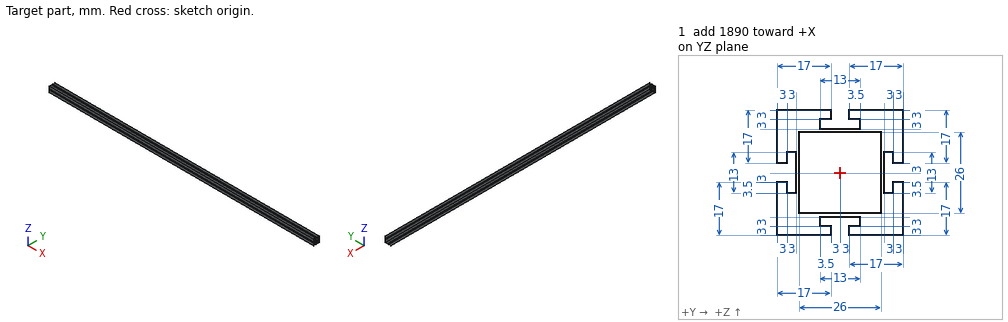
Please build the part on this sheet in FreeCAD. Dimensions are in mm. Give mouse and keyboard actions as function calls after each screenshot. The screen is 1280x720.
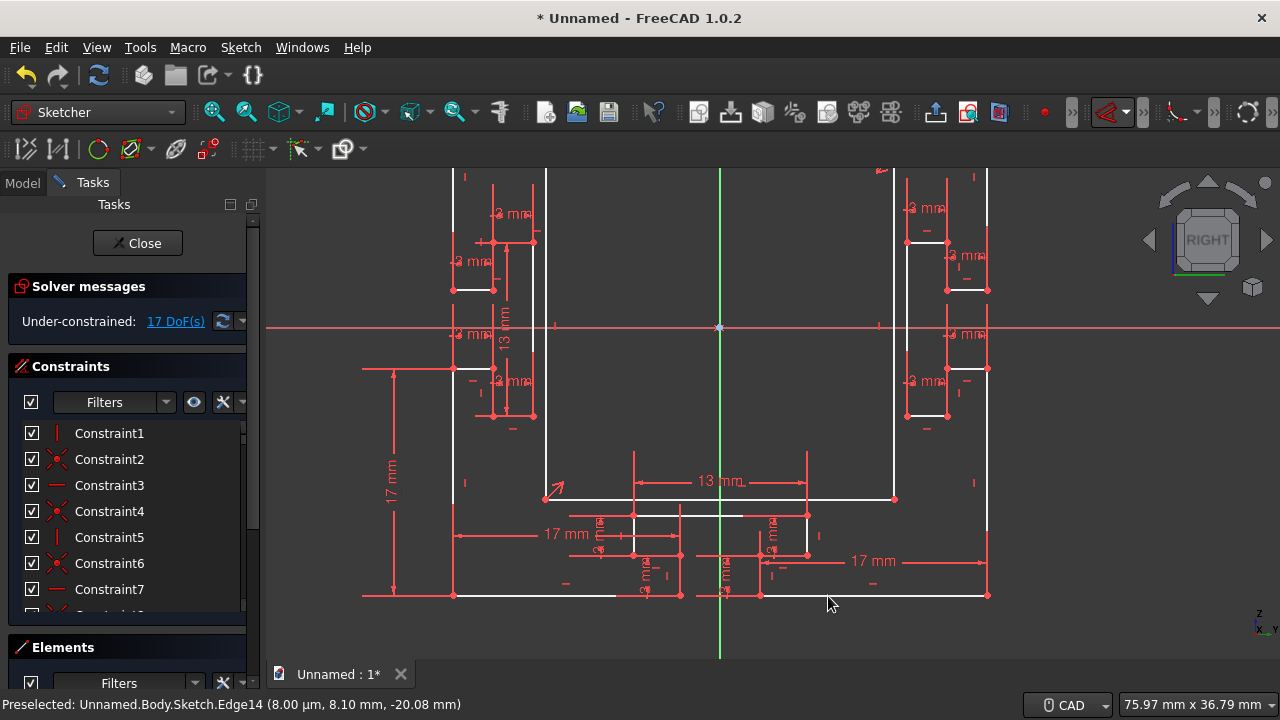
click(987, 528)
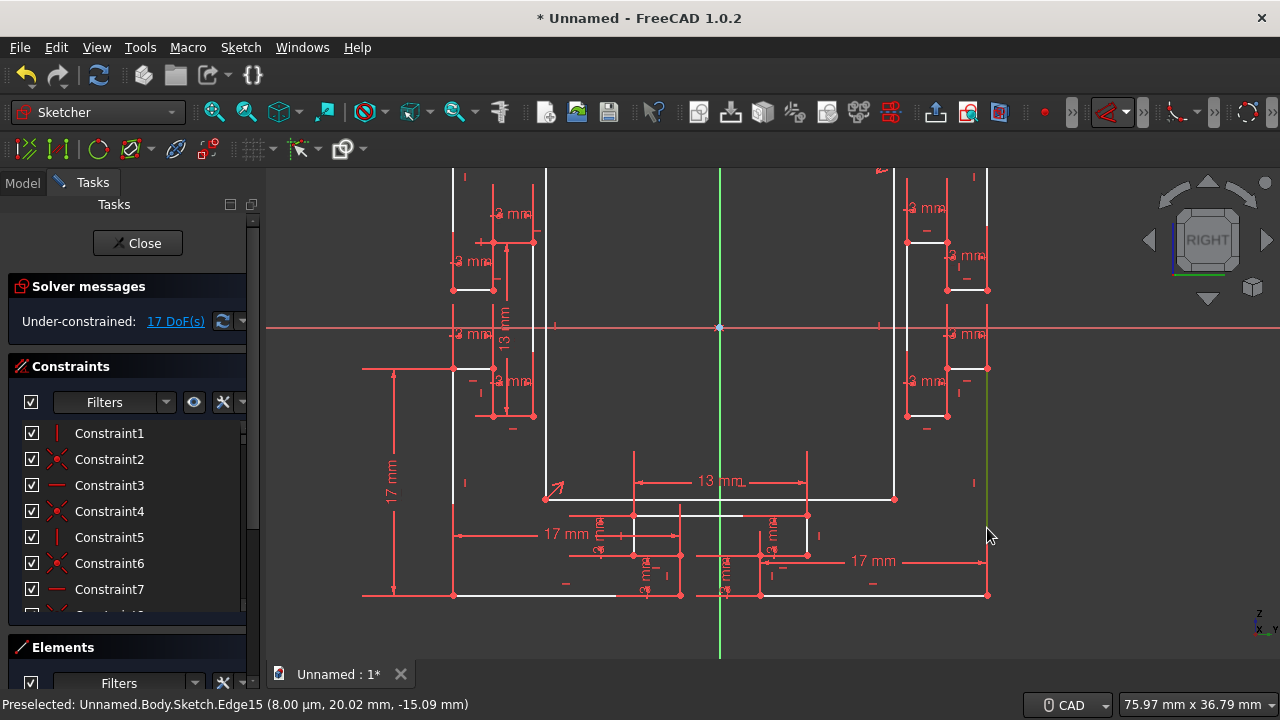
click(1128, 112)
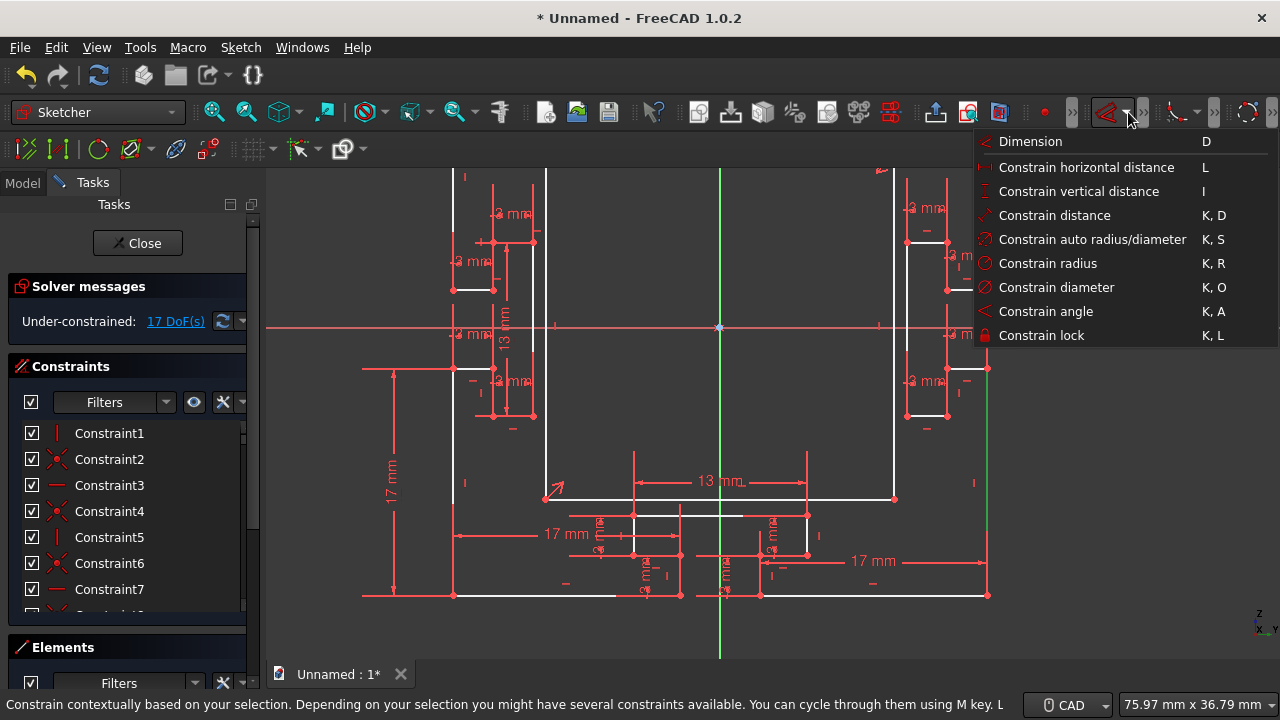
click(1126, 191)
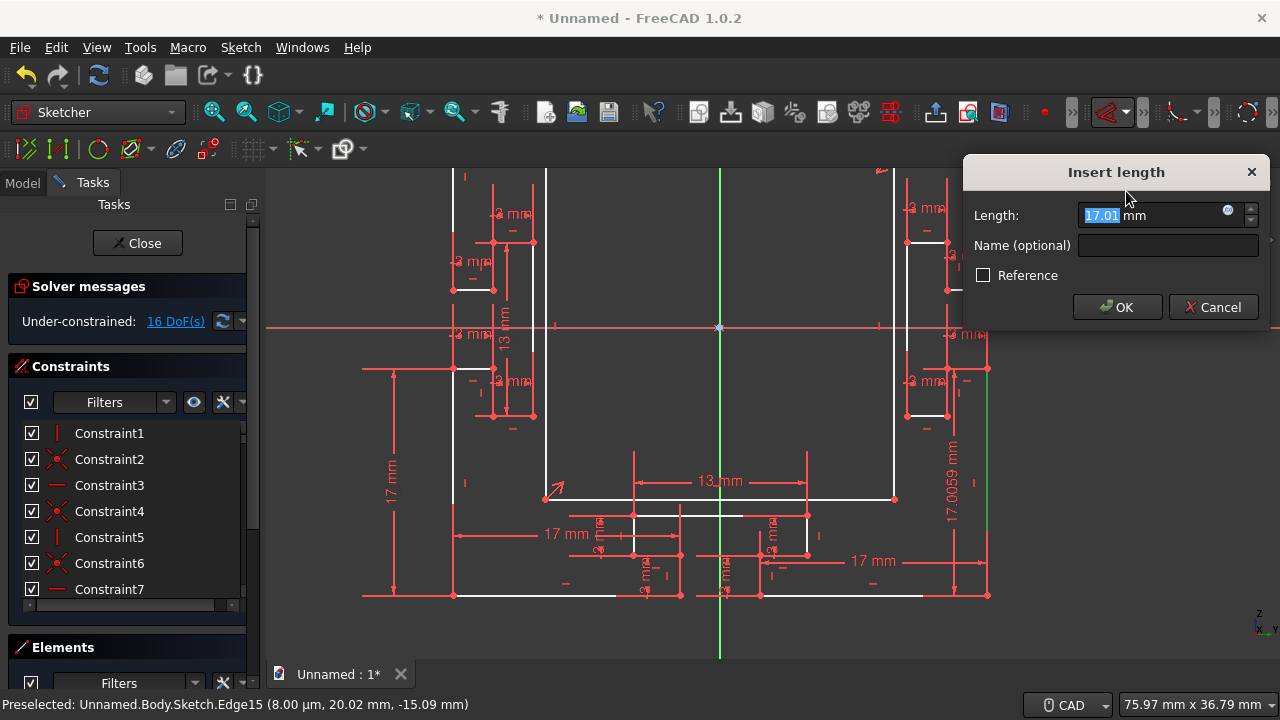
text(17)
key(Return)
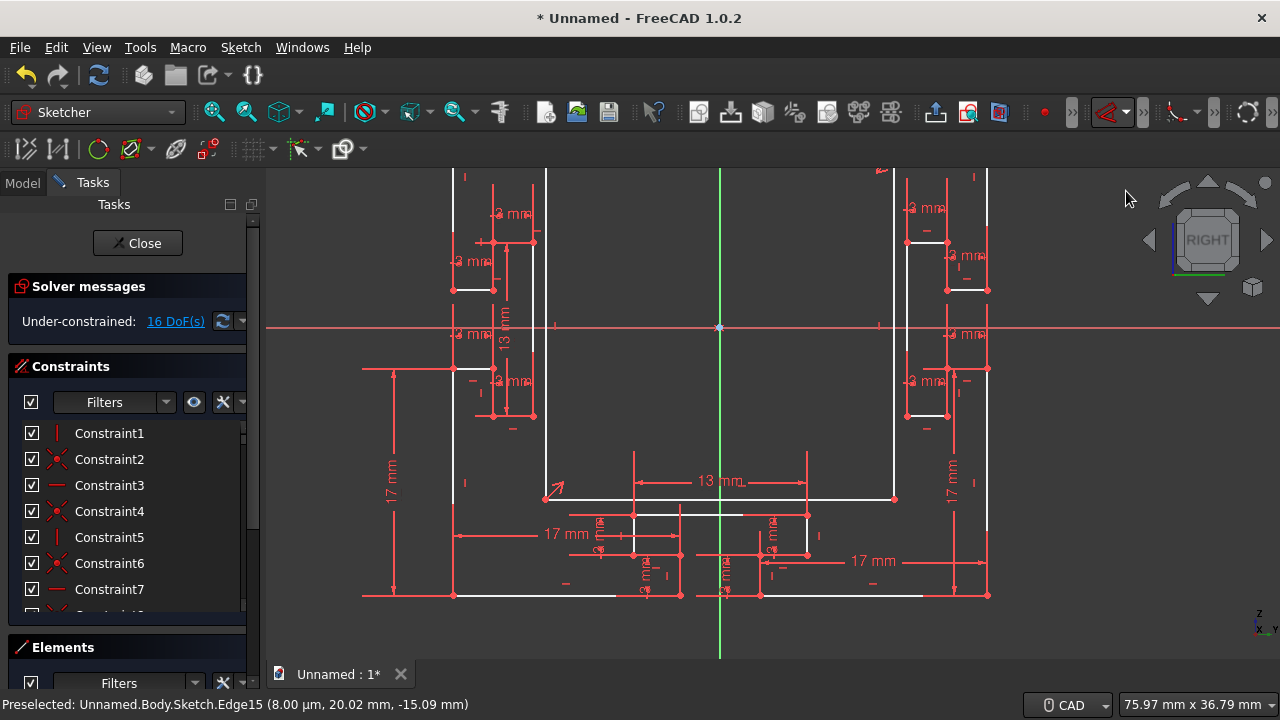
click(907, 364)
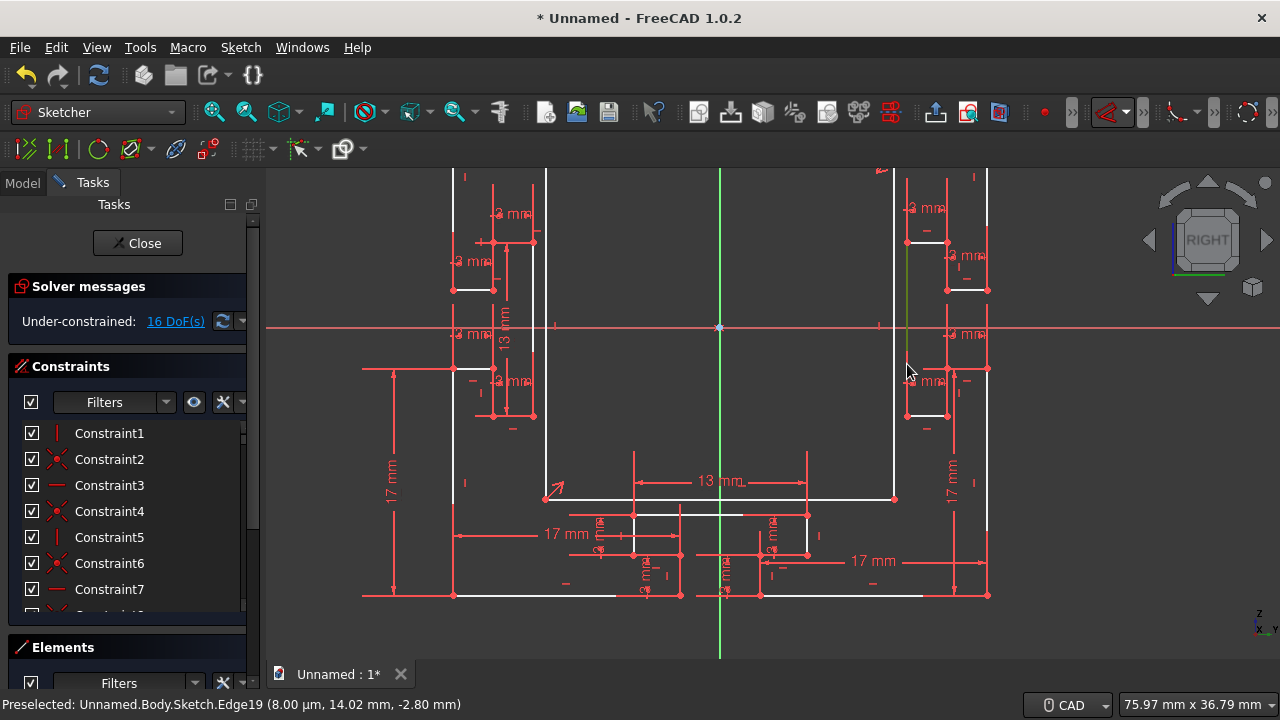
click(1128, 112)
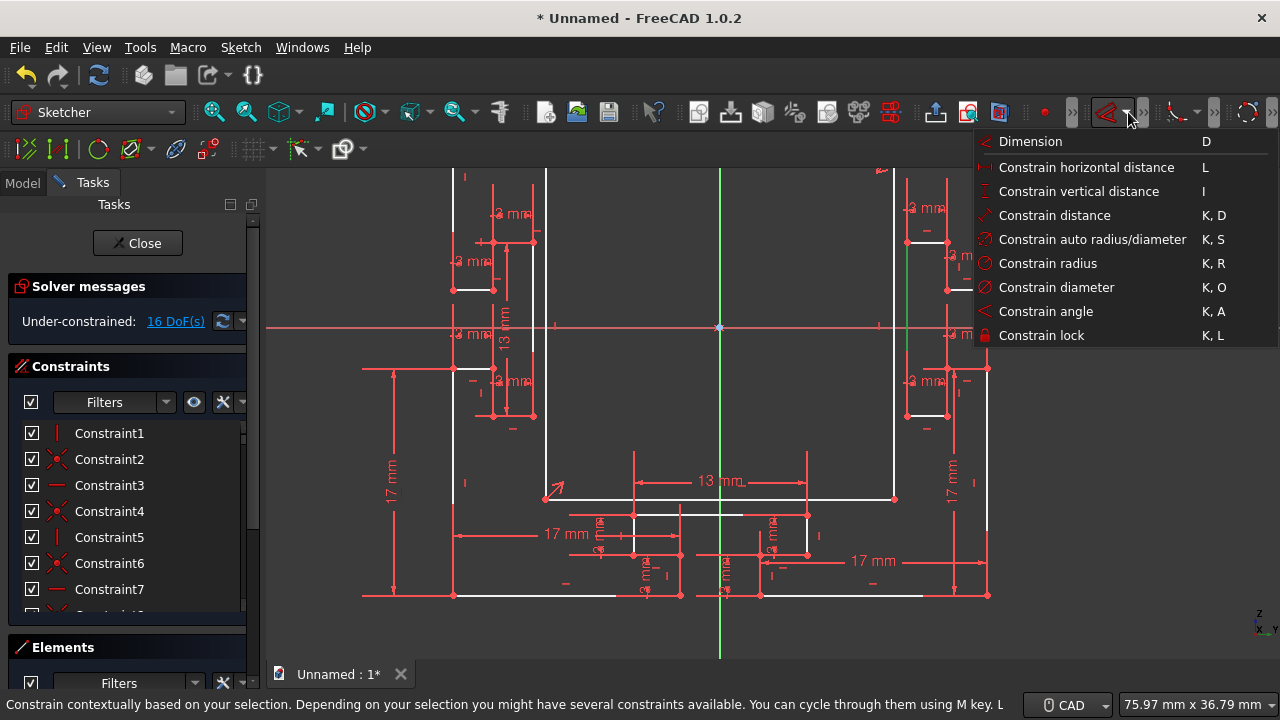
click(1126, 191)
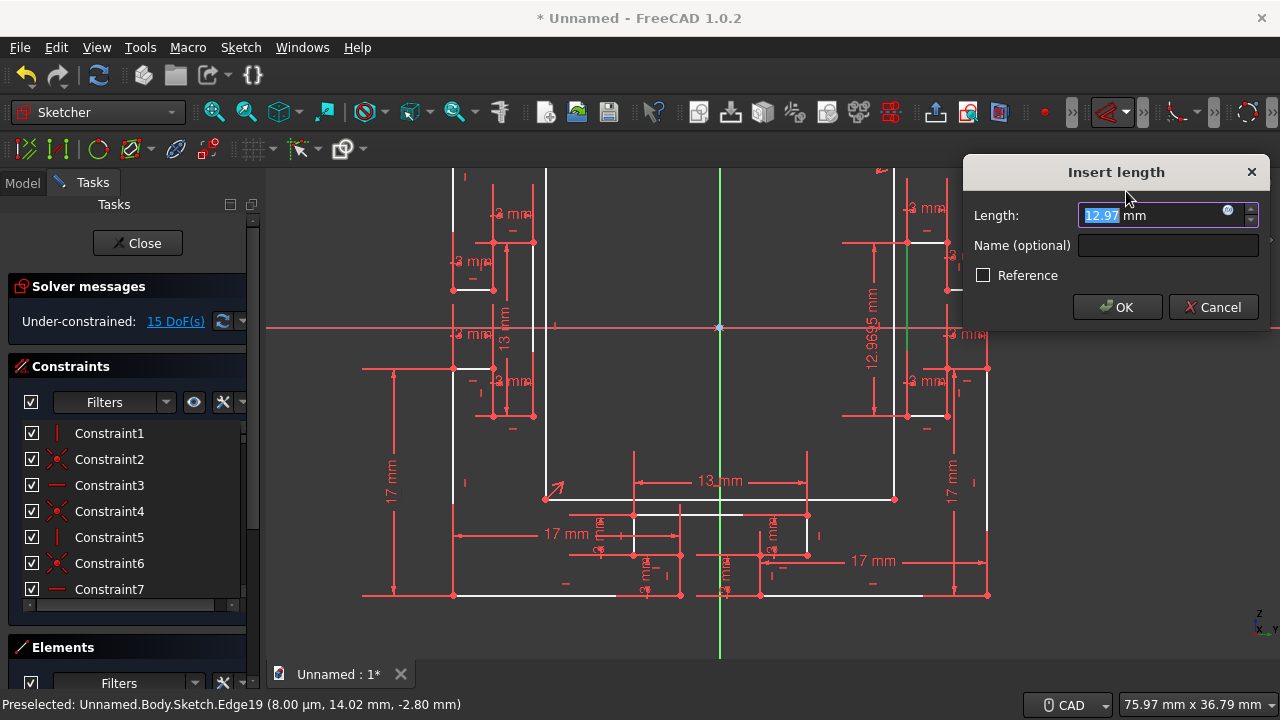
text(13)
key(Return)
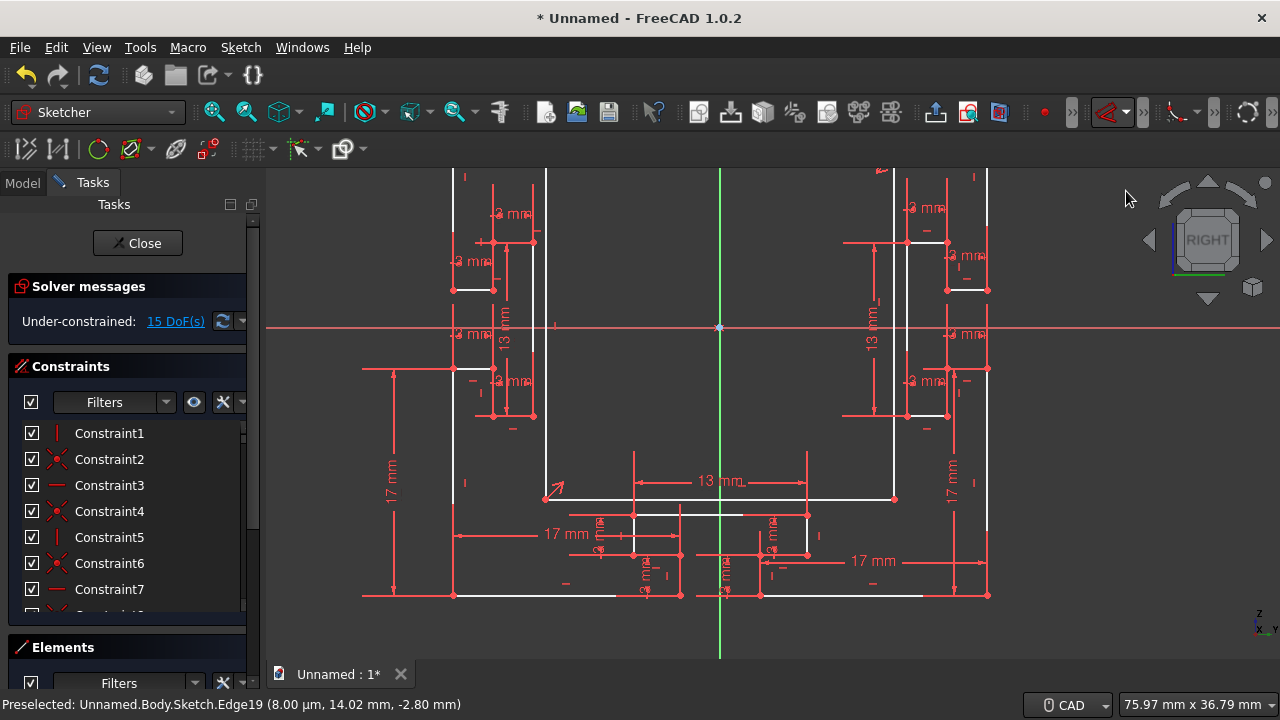
click(987, 222)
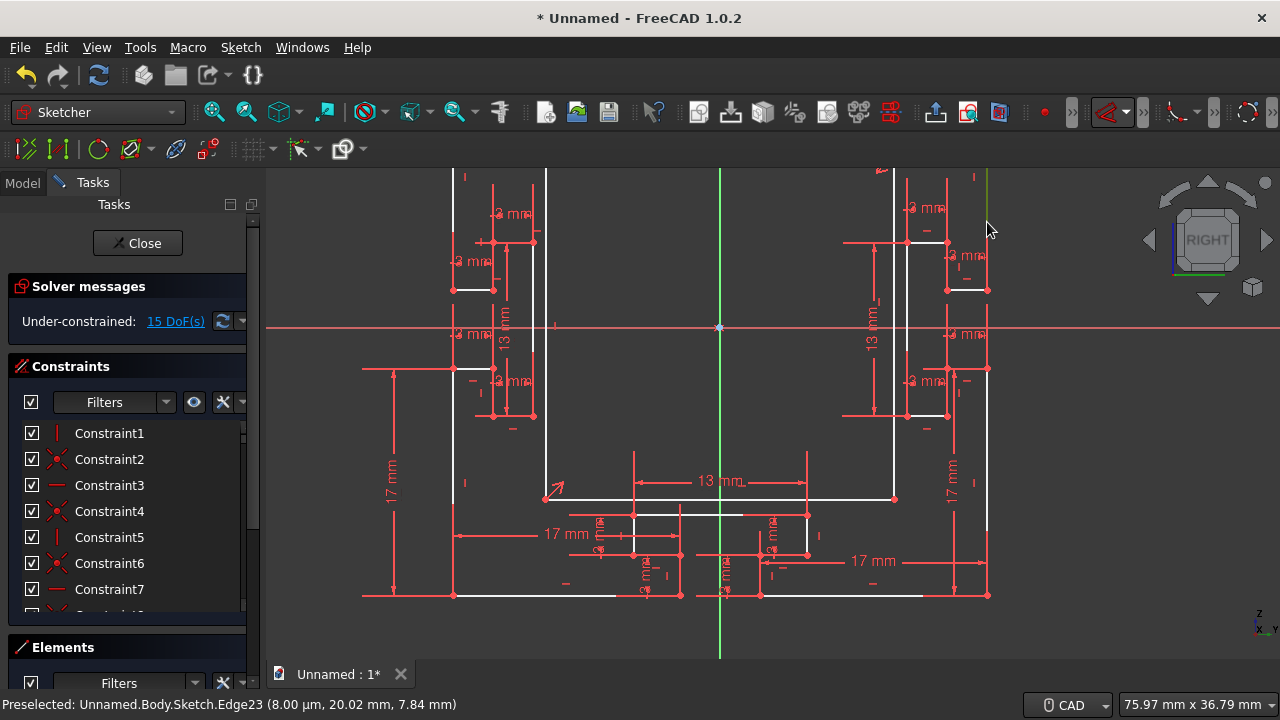
key(i)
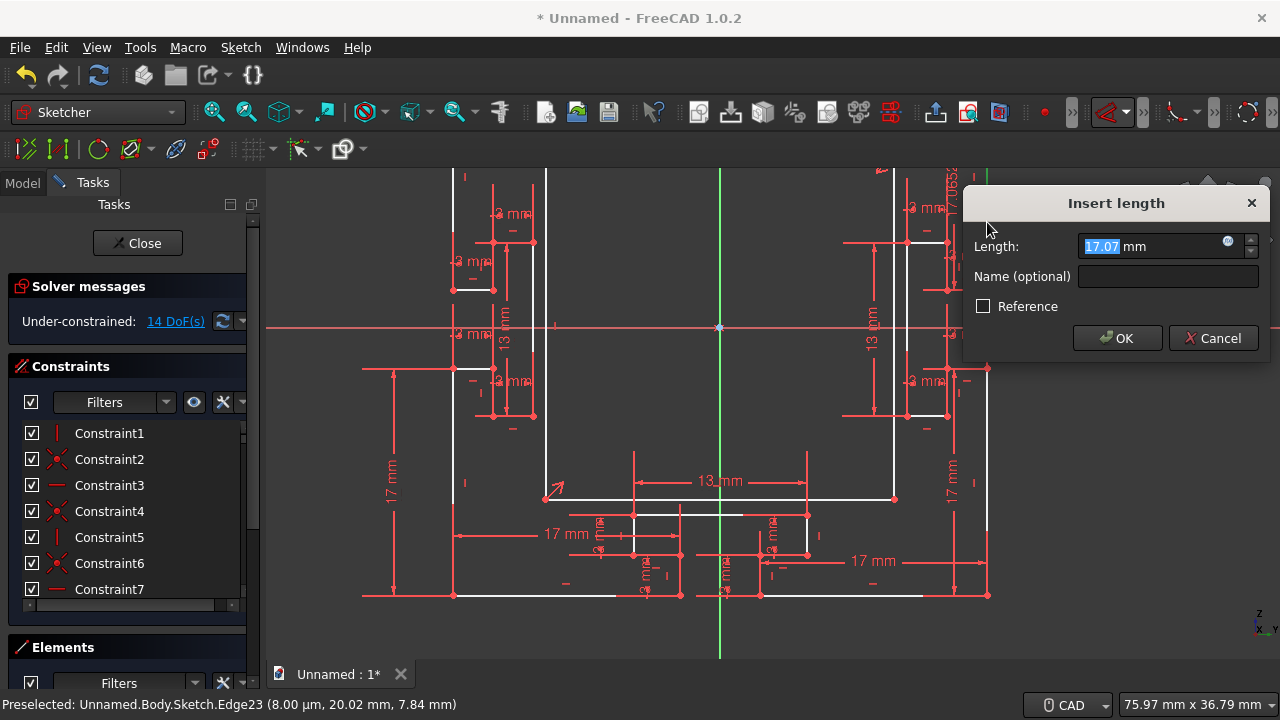
text(17)
key(Return)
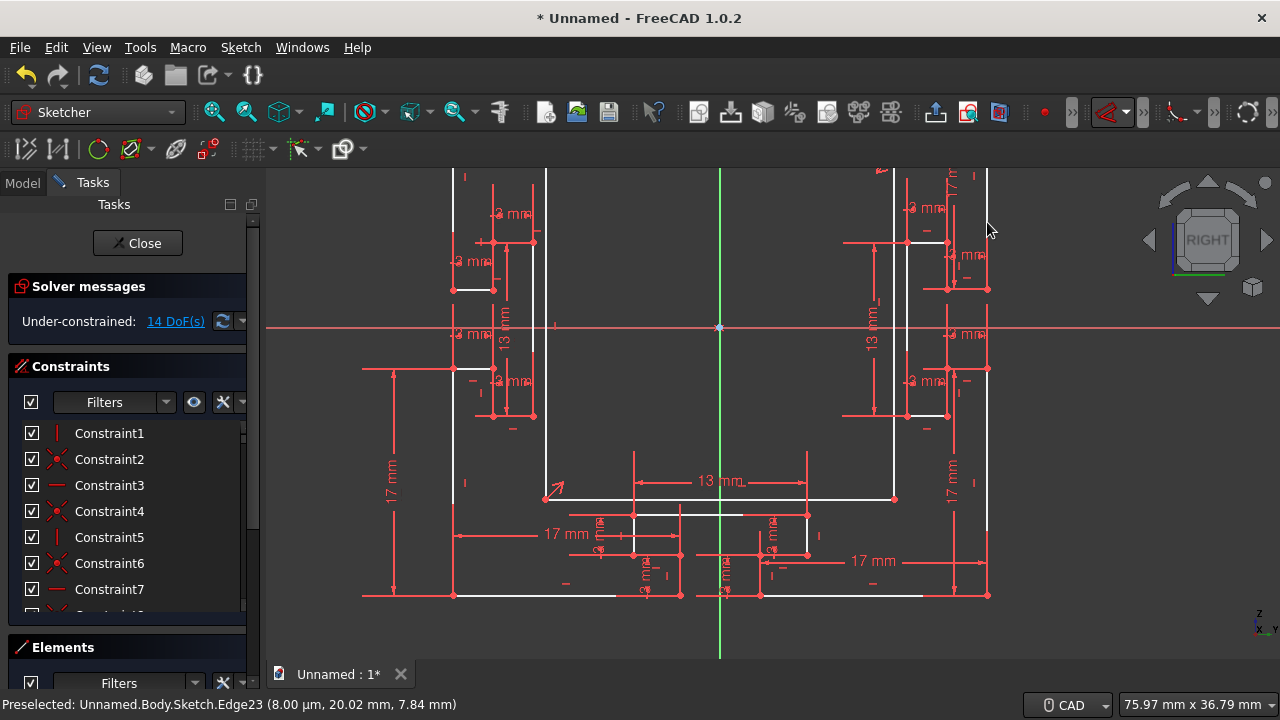
scroll(686, 518, down, 3)